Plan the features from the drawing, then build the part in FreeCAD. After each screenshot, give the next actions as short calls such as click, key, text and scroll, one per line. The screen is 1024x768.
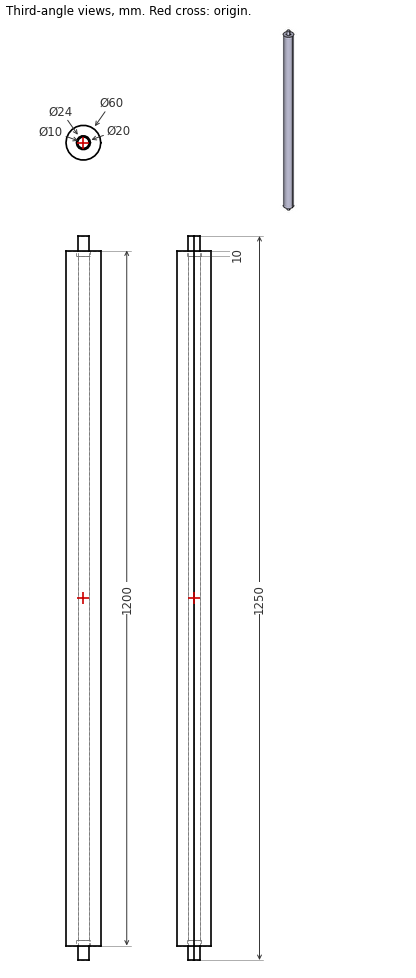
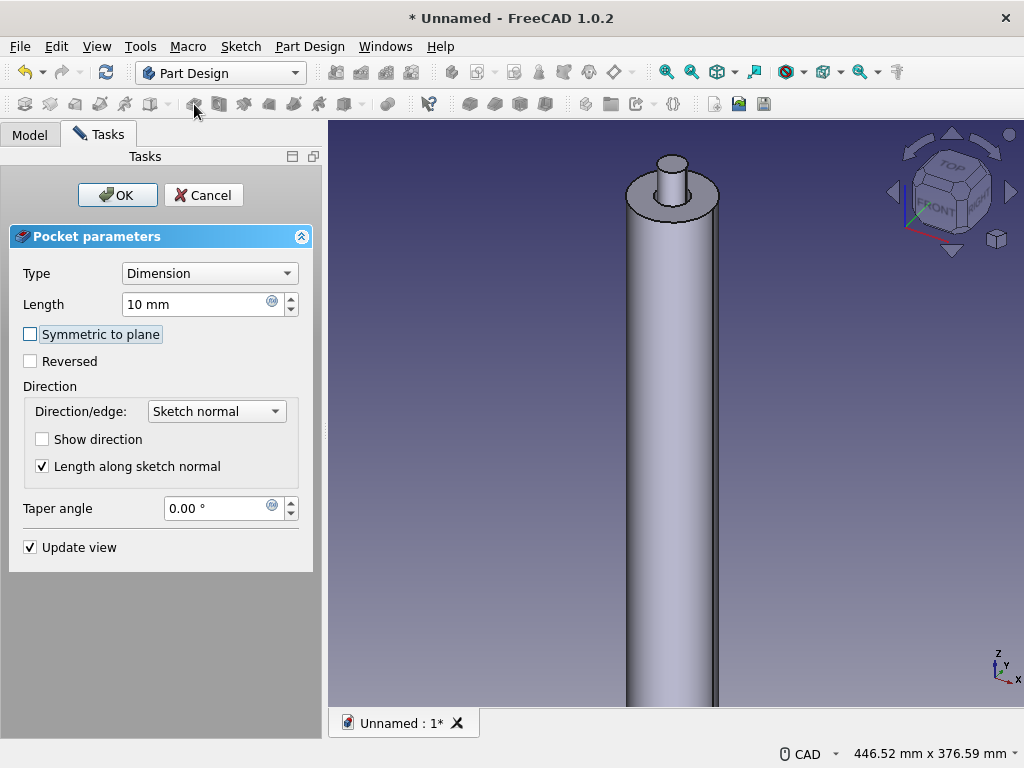
click(118, 195)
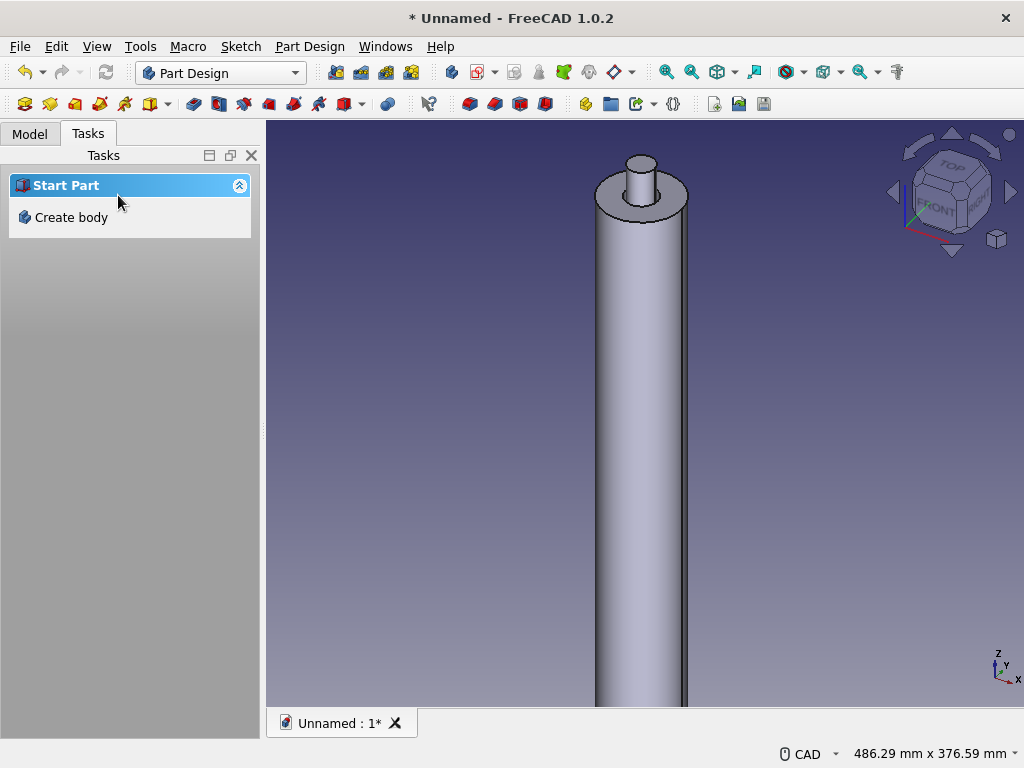
key(v)
key(f)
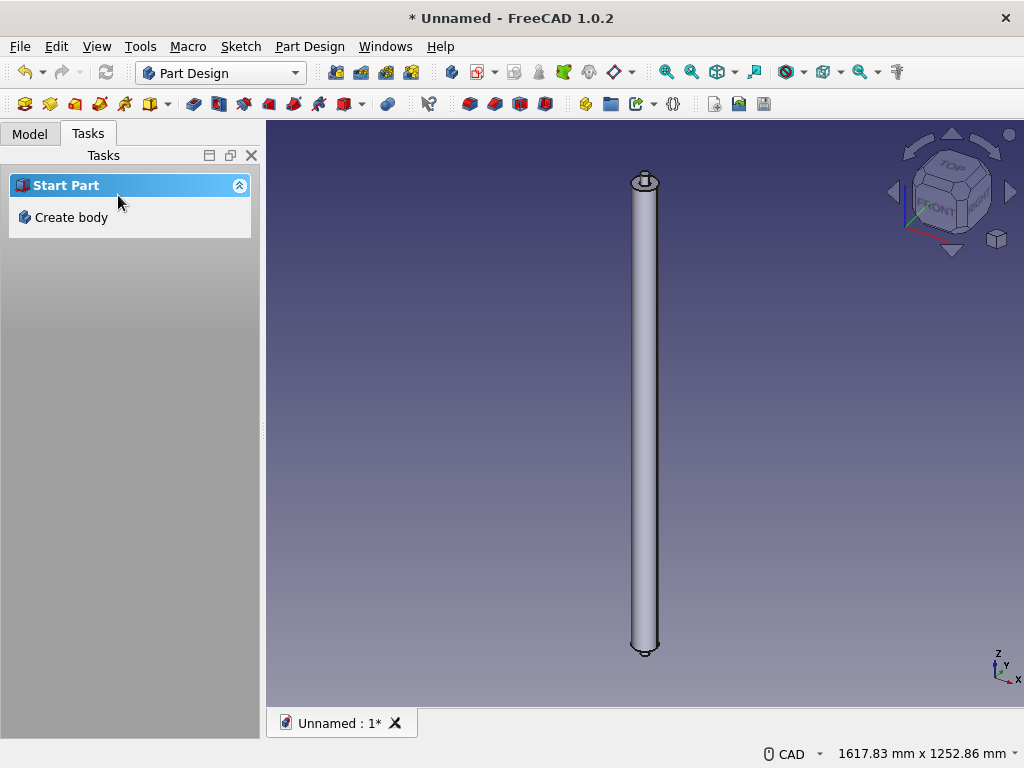
click(30, 134)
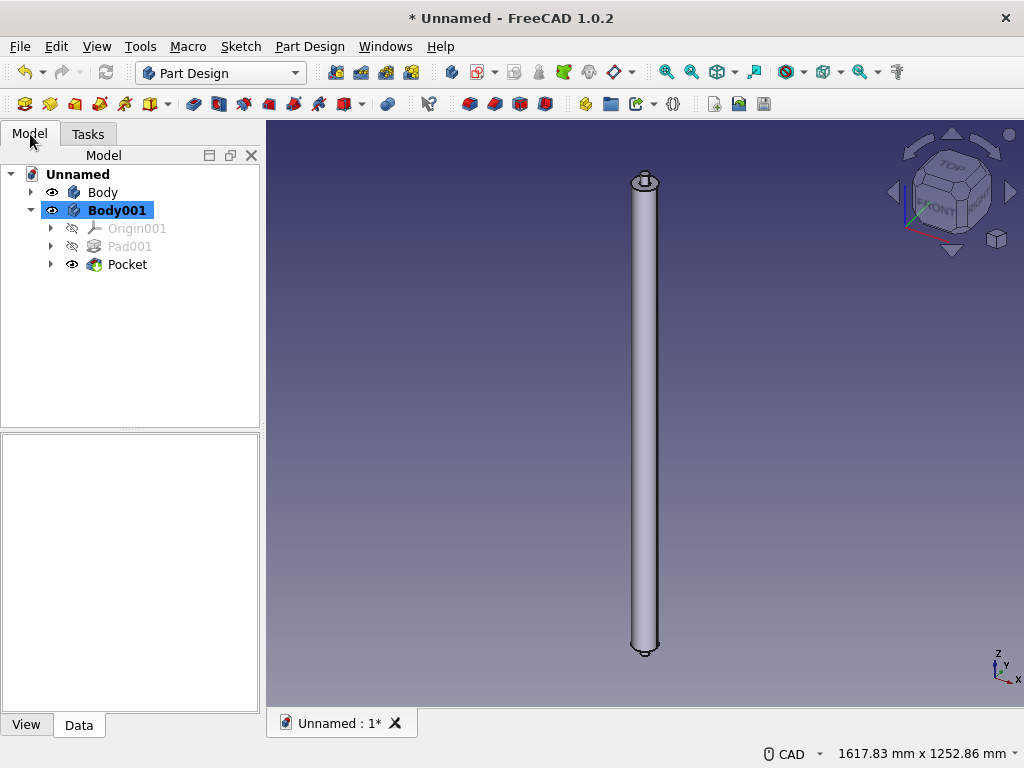
click(117, 264)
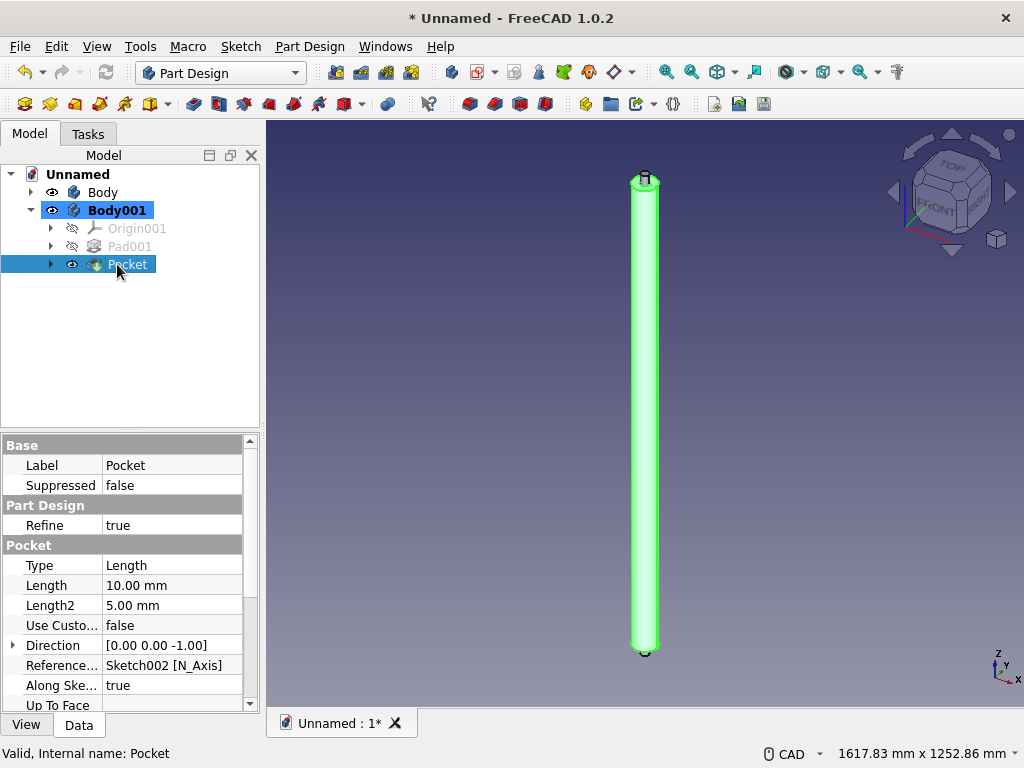
click(336, 72)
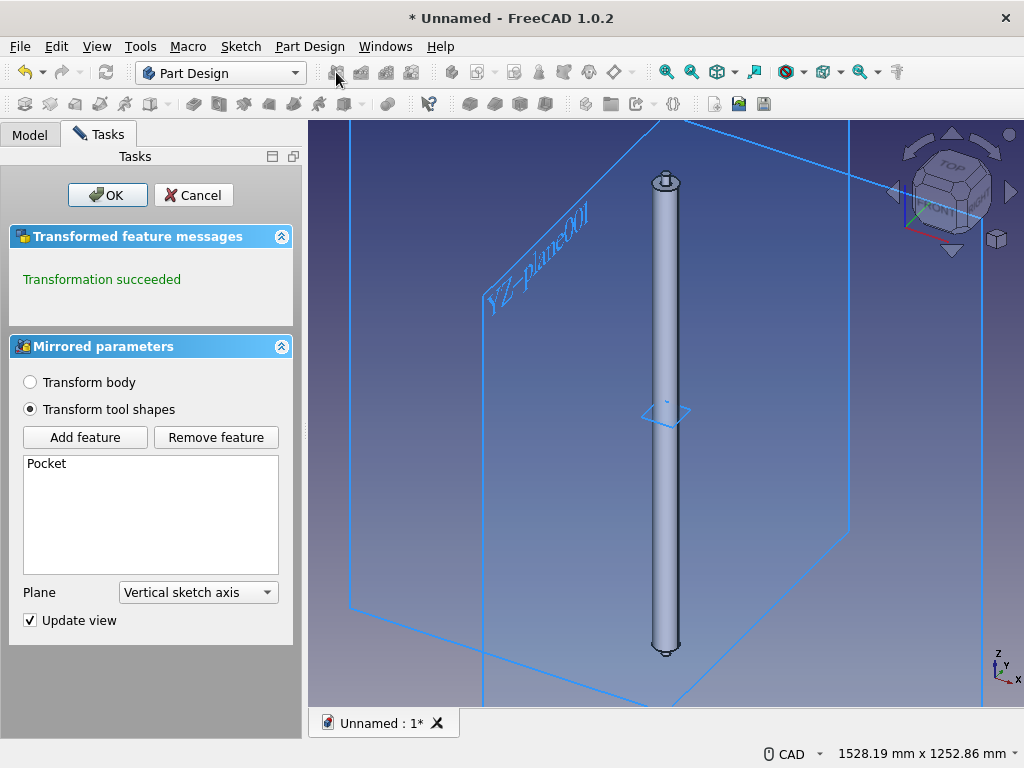
click(199, 592)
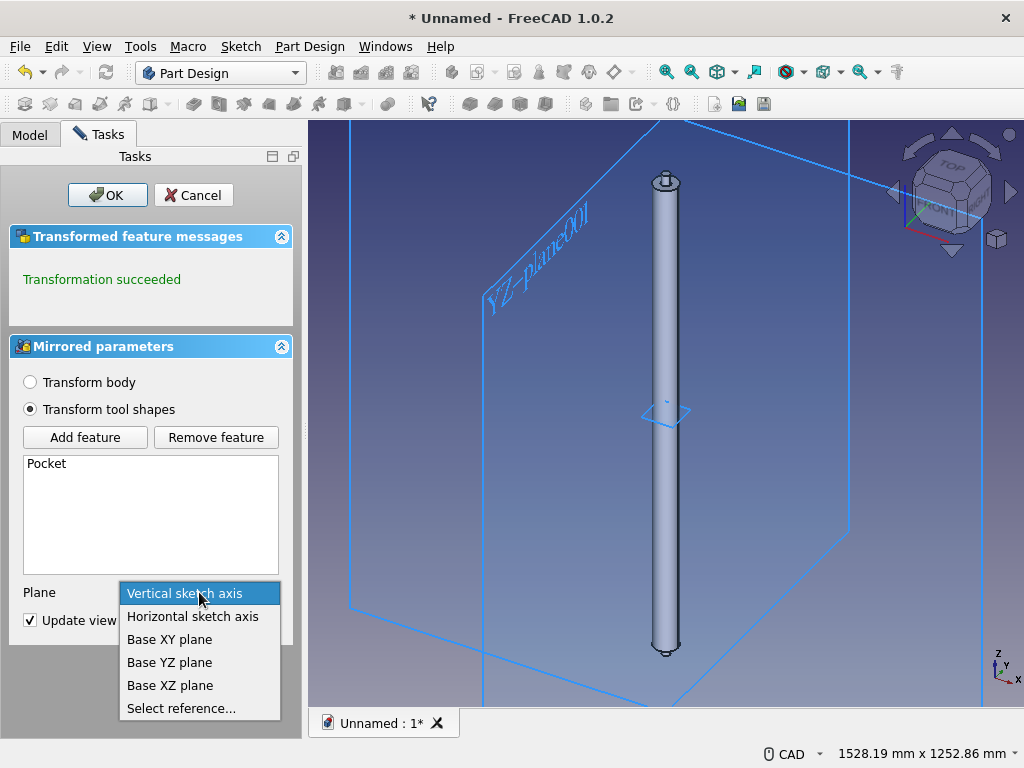
click(198, 640)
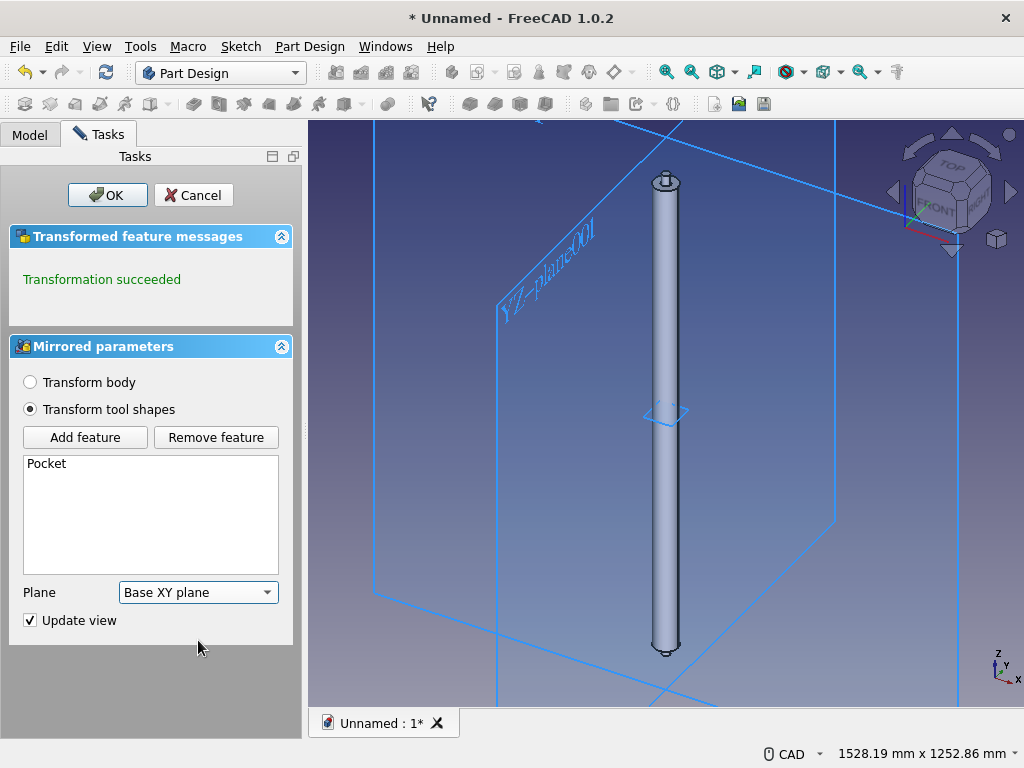
click(108, 195)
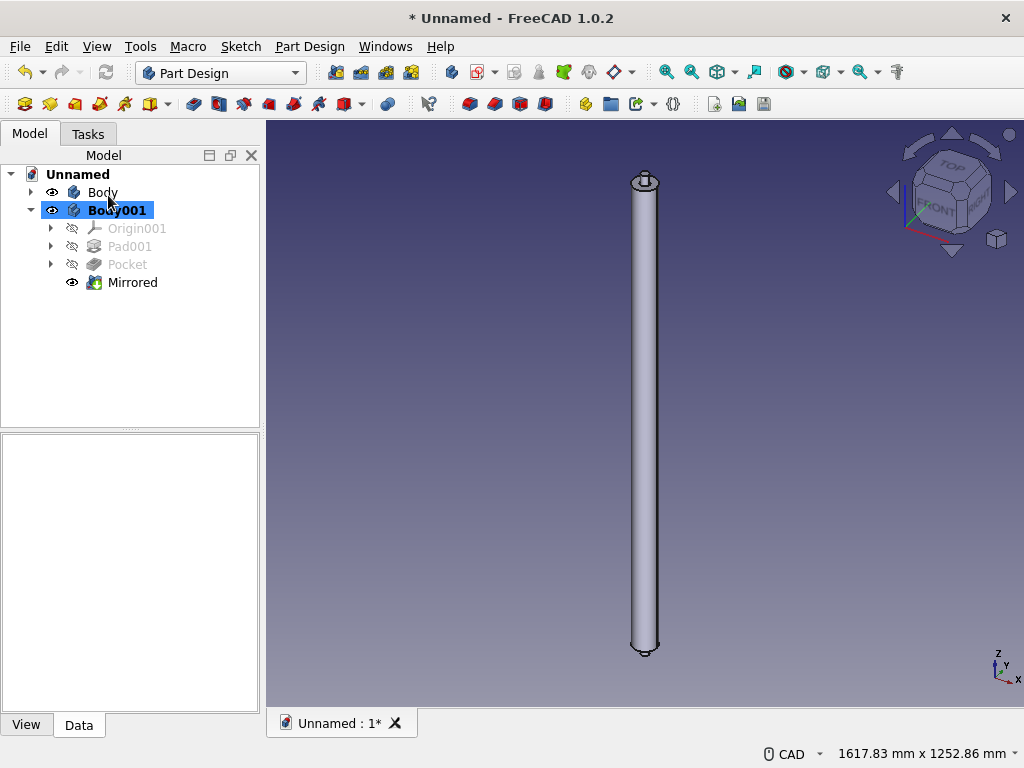
key(0)